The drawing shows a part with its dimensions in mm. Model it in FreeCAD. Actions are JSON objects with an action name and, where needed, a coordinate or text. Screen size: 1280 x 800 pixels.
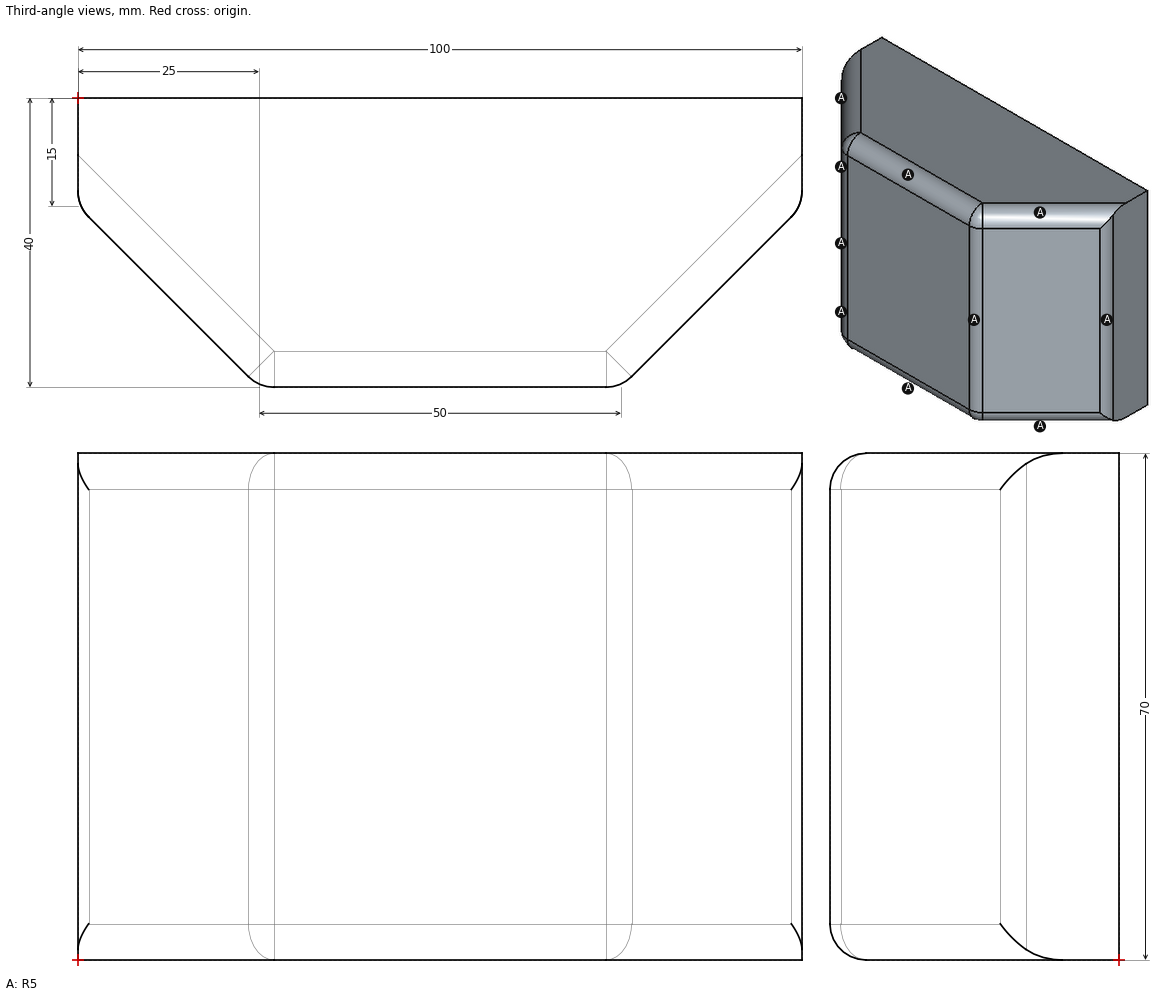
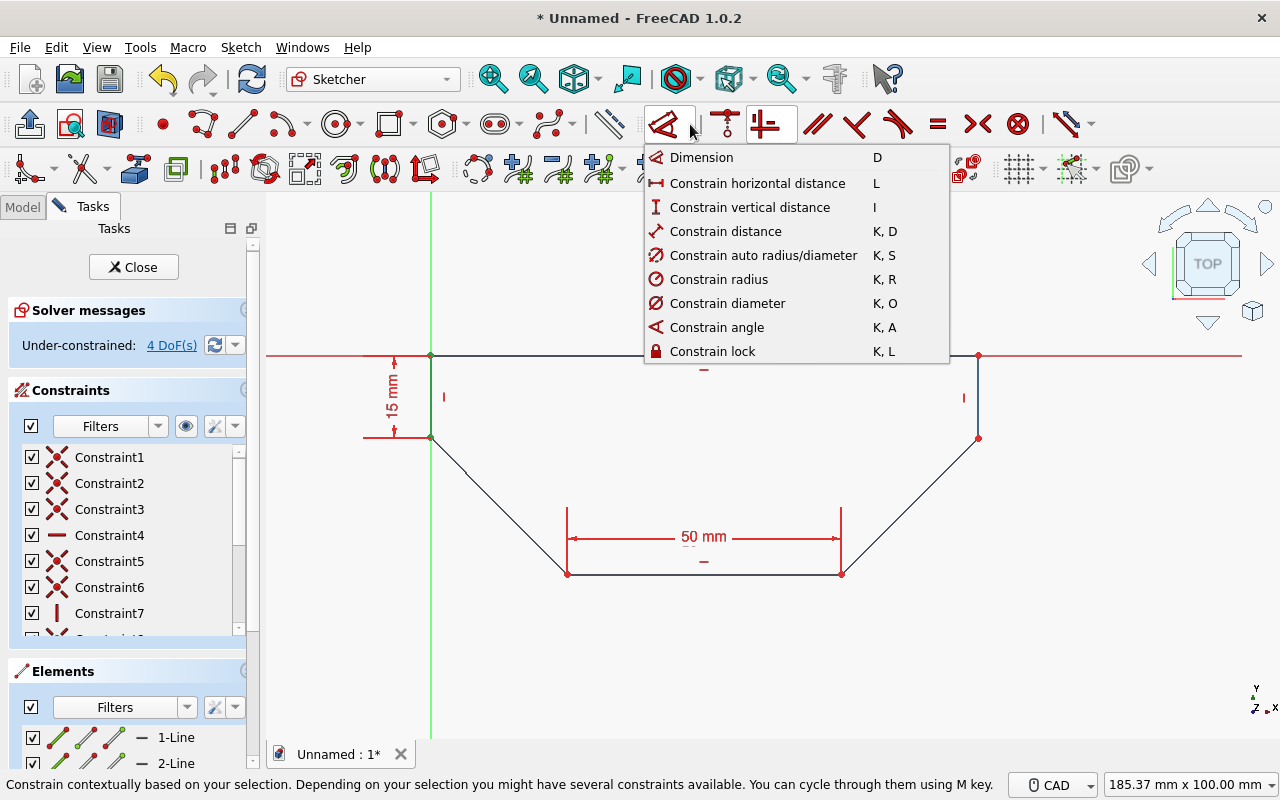
{"action": "left_click", "coordinate": [797, 207]}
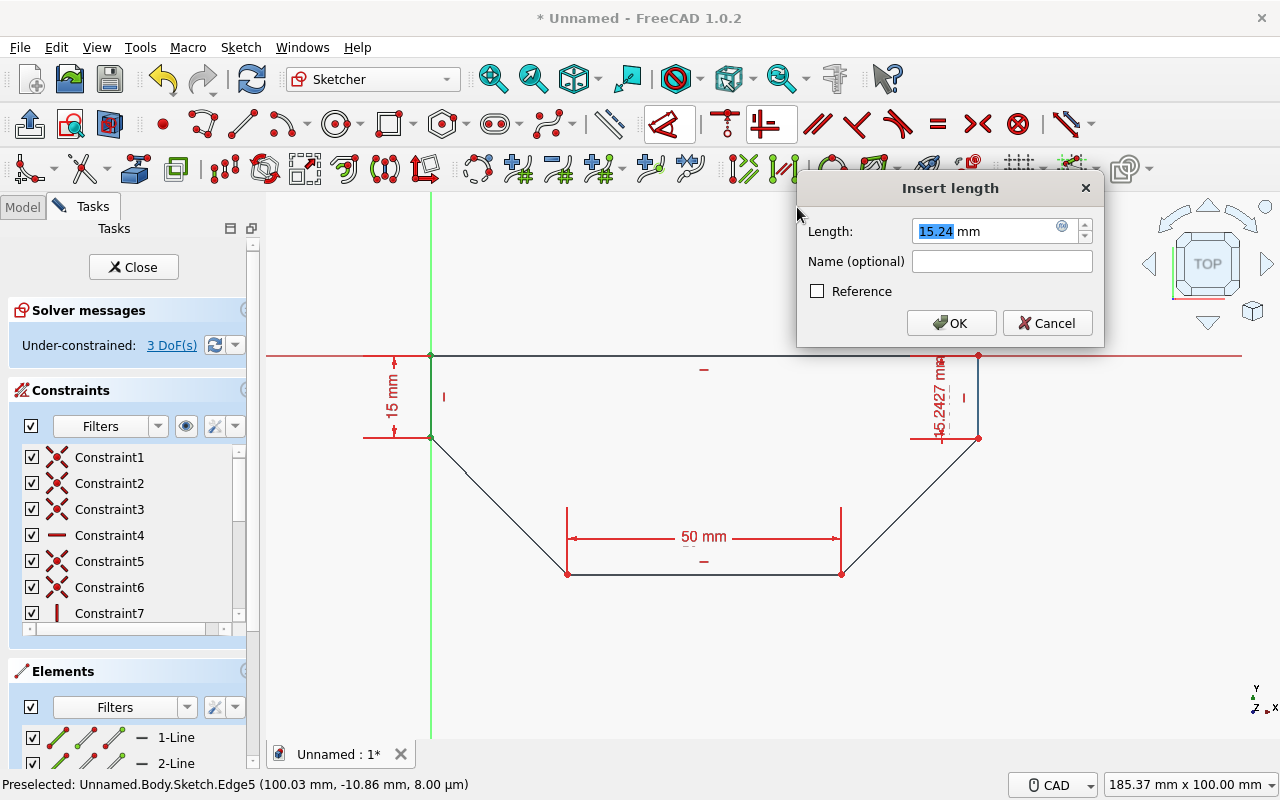
{"action": "type", "text": "15"}
{"action": "key", "text": "Return"}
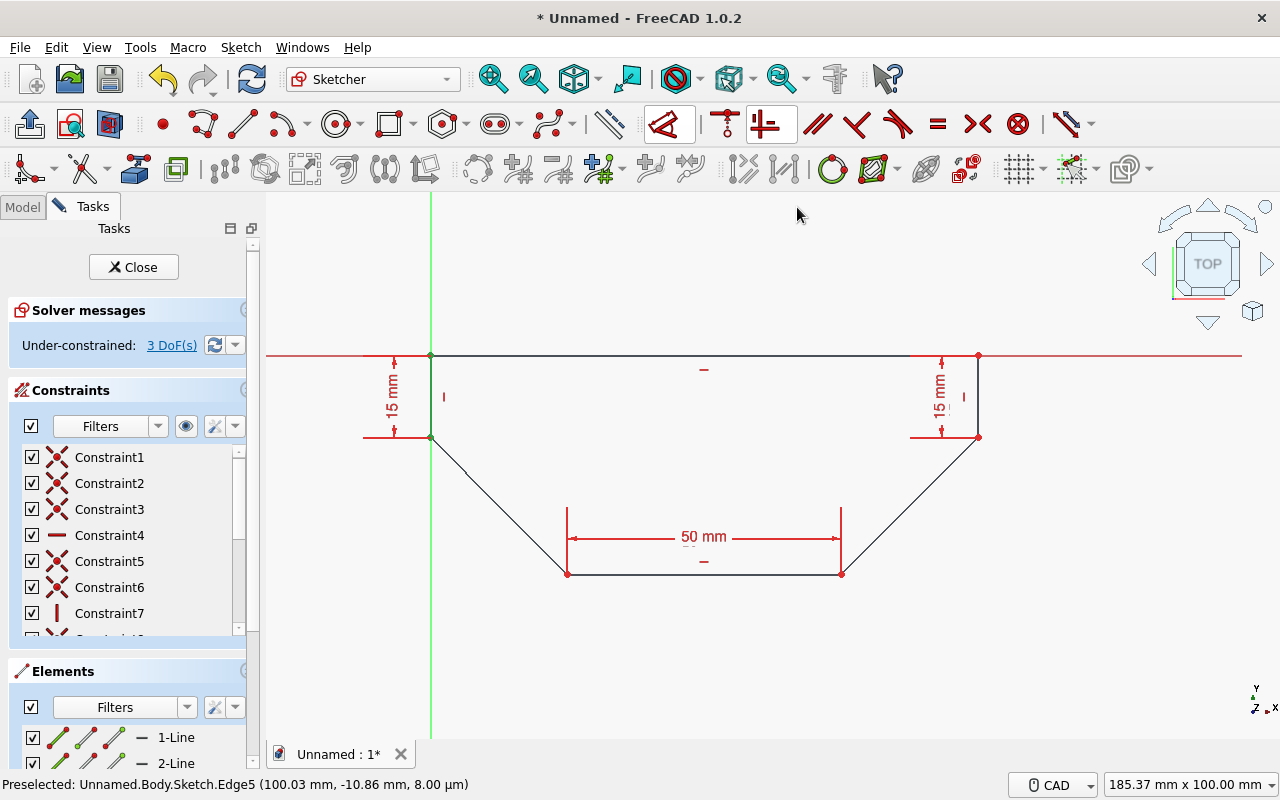
{"action": "left_click", "coordinate": [814, 356]}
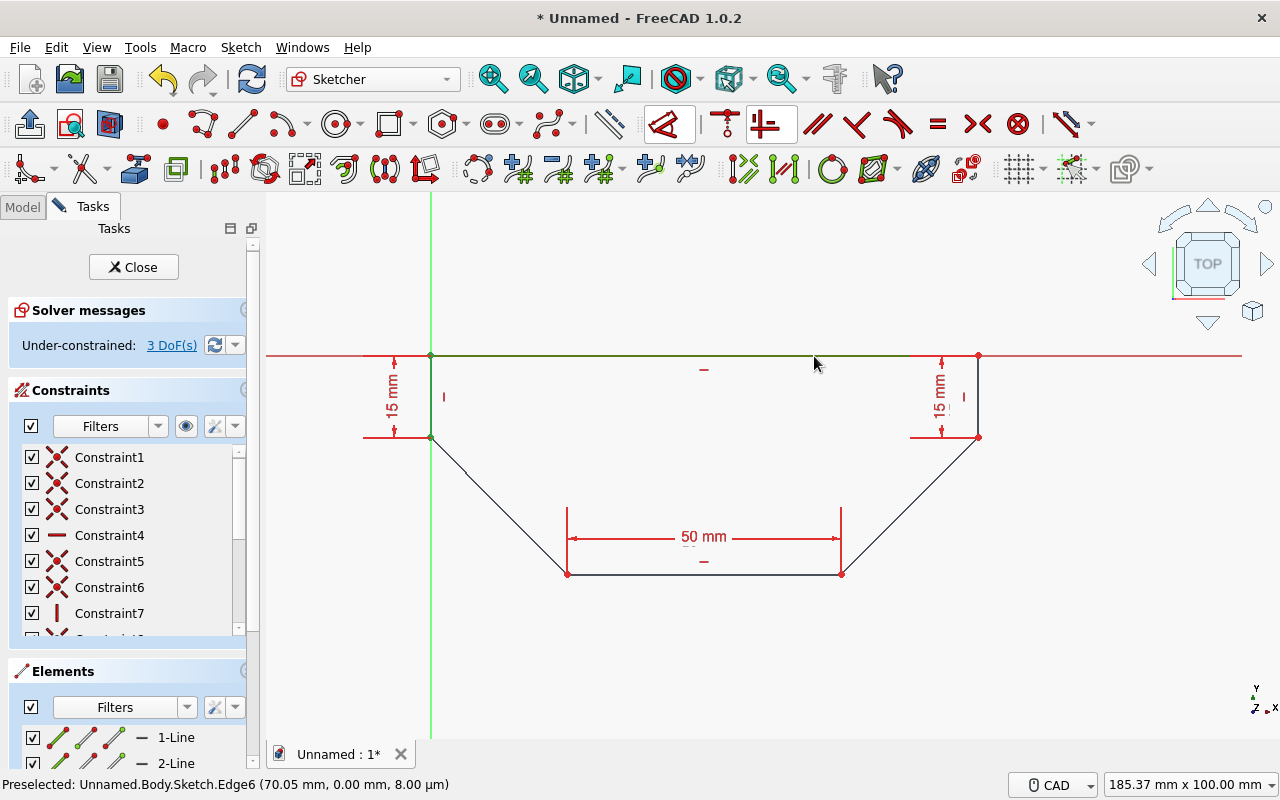
{"action": "key", "text": "l"}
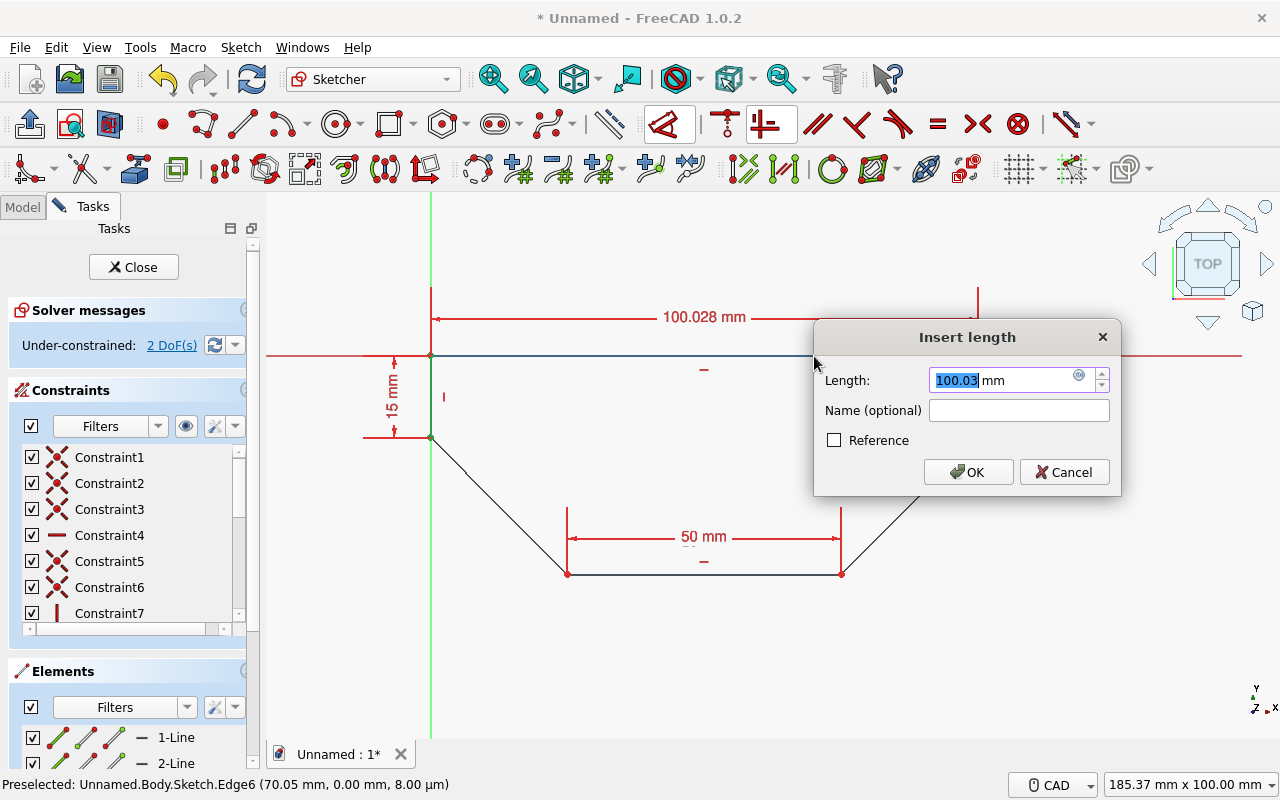
{"action": "type", "text": "100"}
{"action": "key", "text": "Return"}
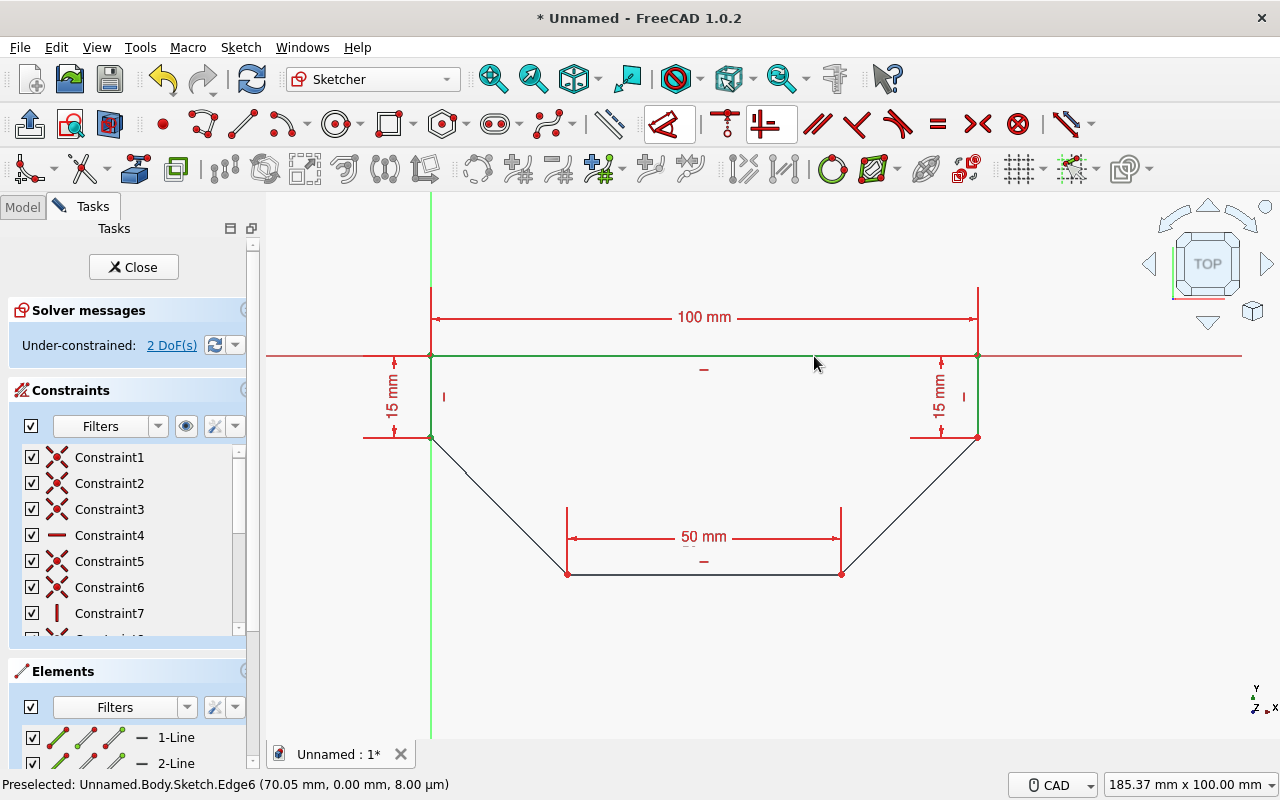
{"action": "left_click", "coordinate": [567, 575]}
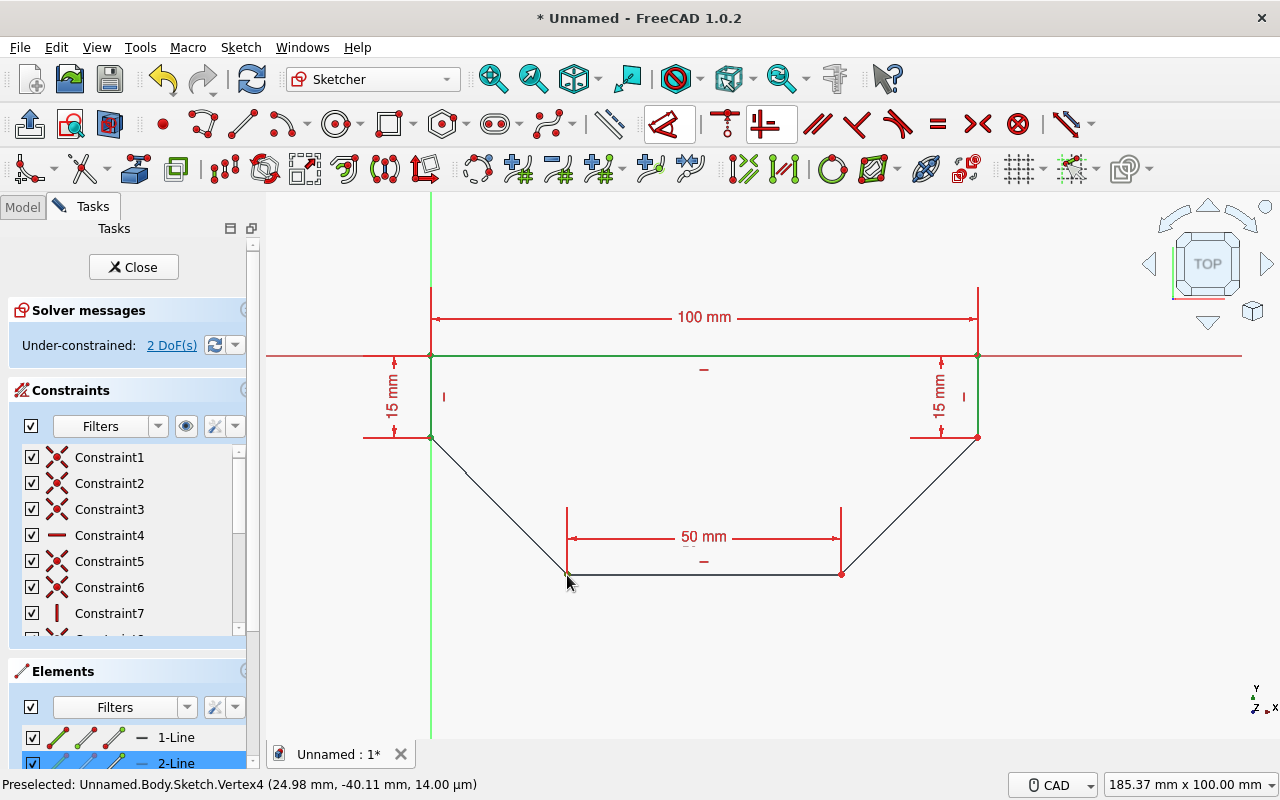
{"action": "key", "text": "l"}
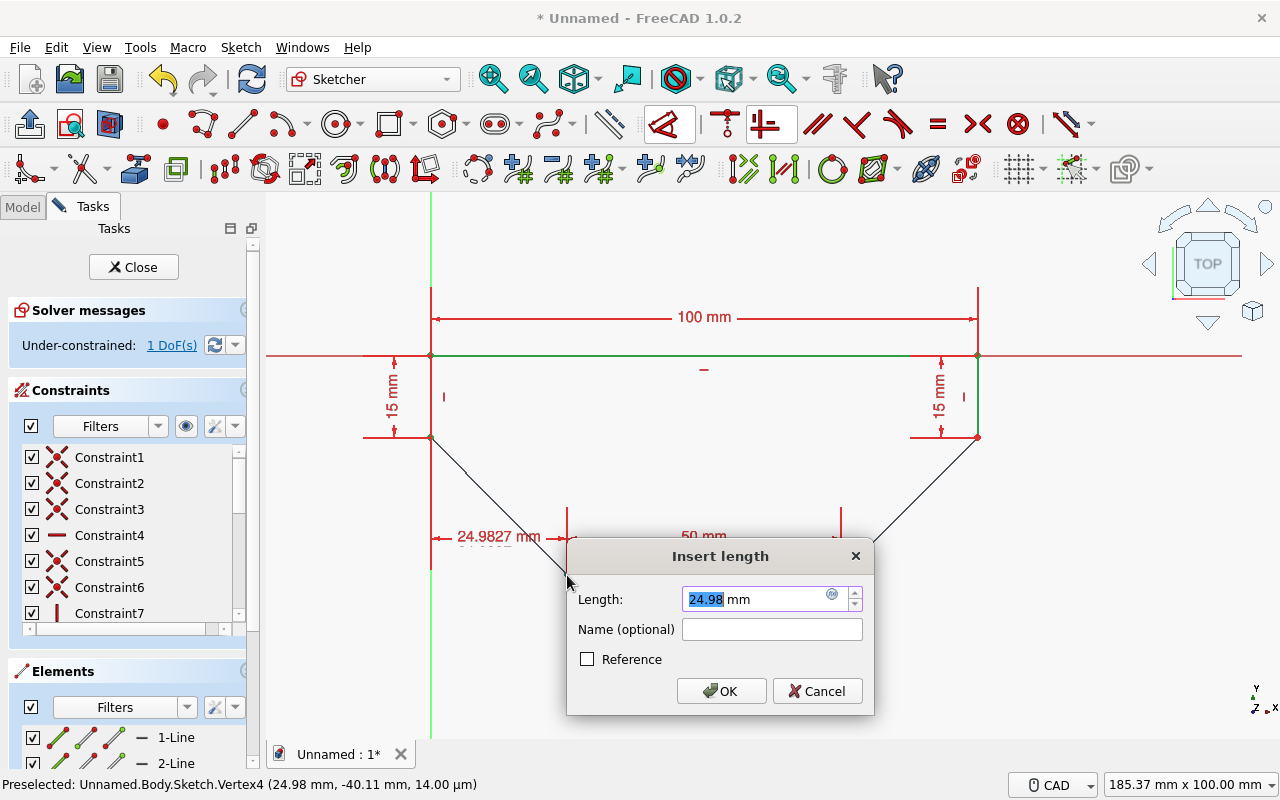
{"action": "type", "text": "25"}
{"action": "key", "text": "Return"}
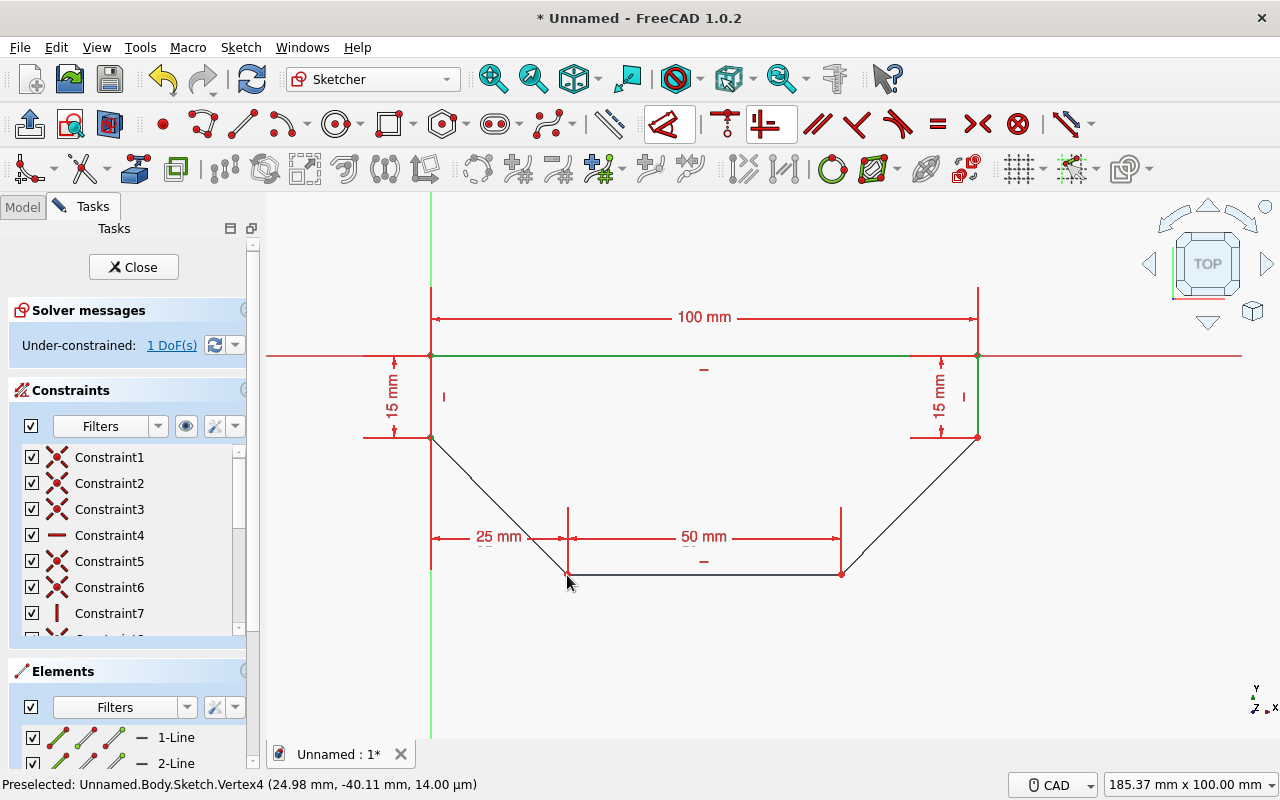
{"action": "left_click", "coordinate": [568, 575]}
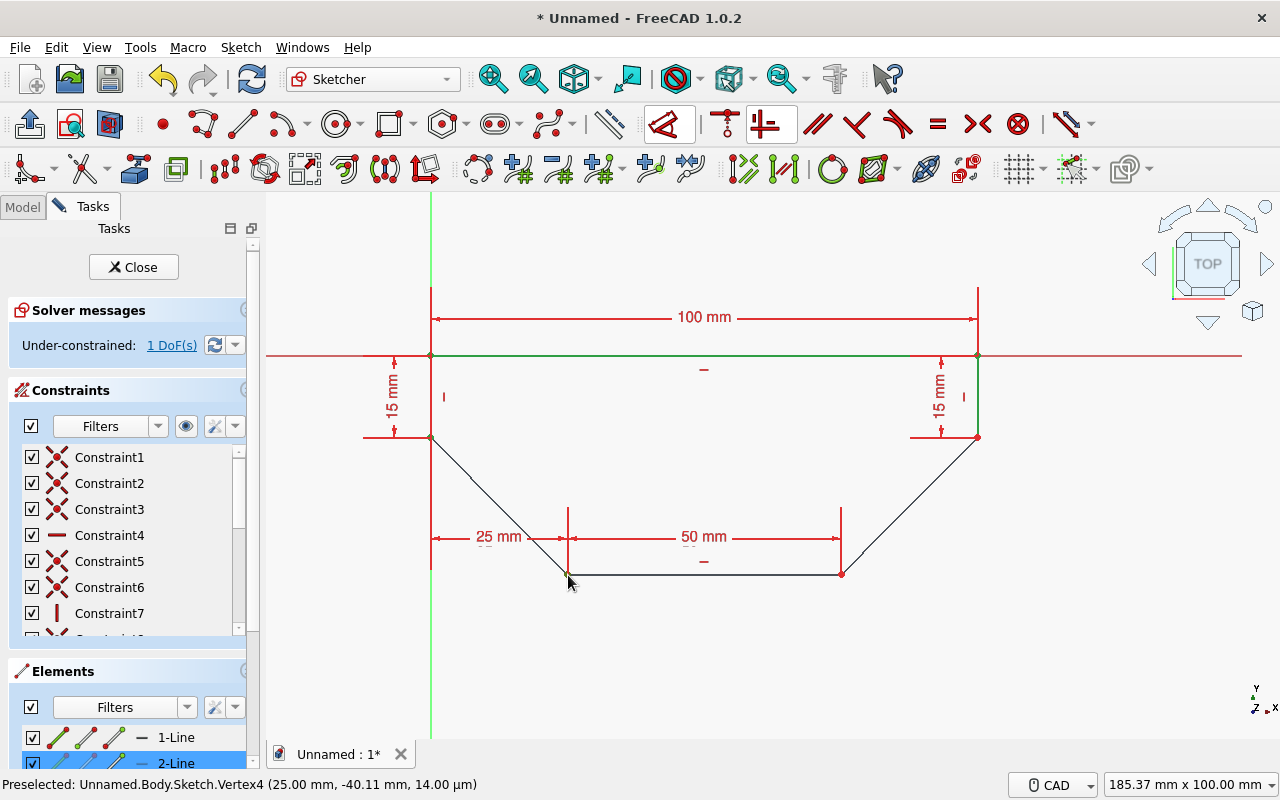
{"action": "key", "text": "i"}